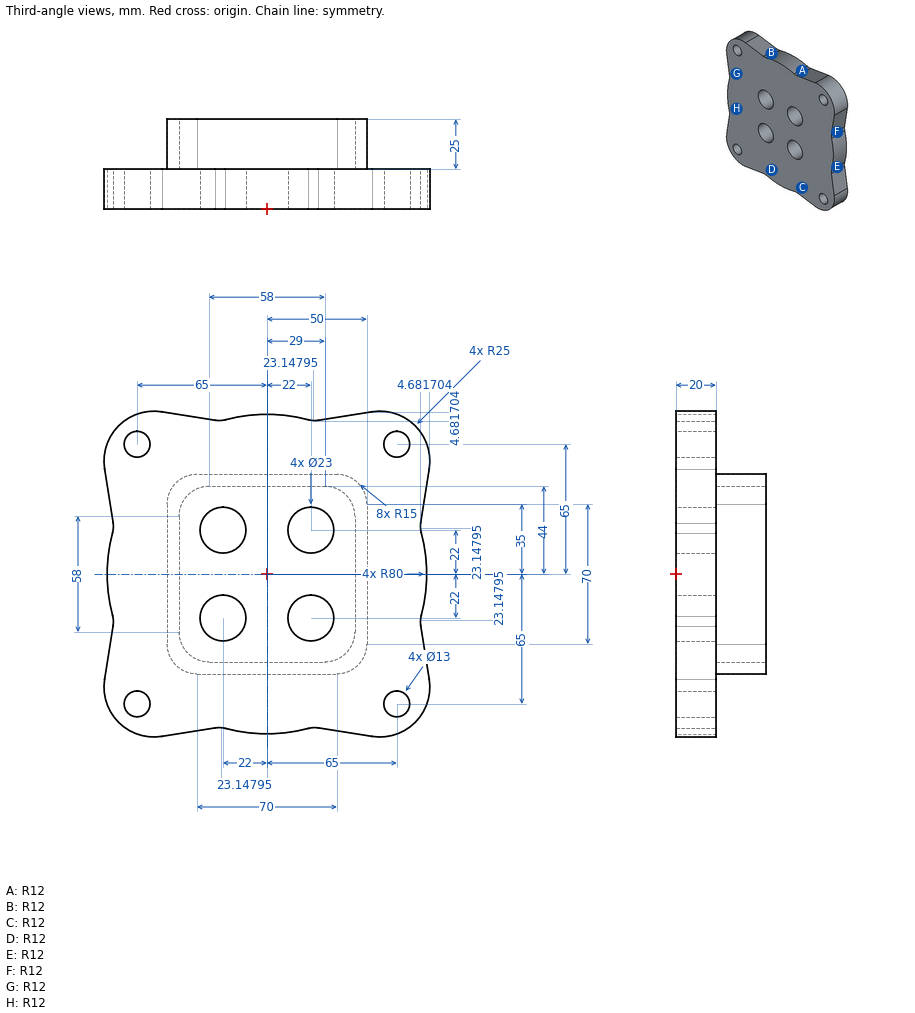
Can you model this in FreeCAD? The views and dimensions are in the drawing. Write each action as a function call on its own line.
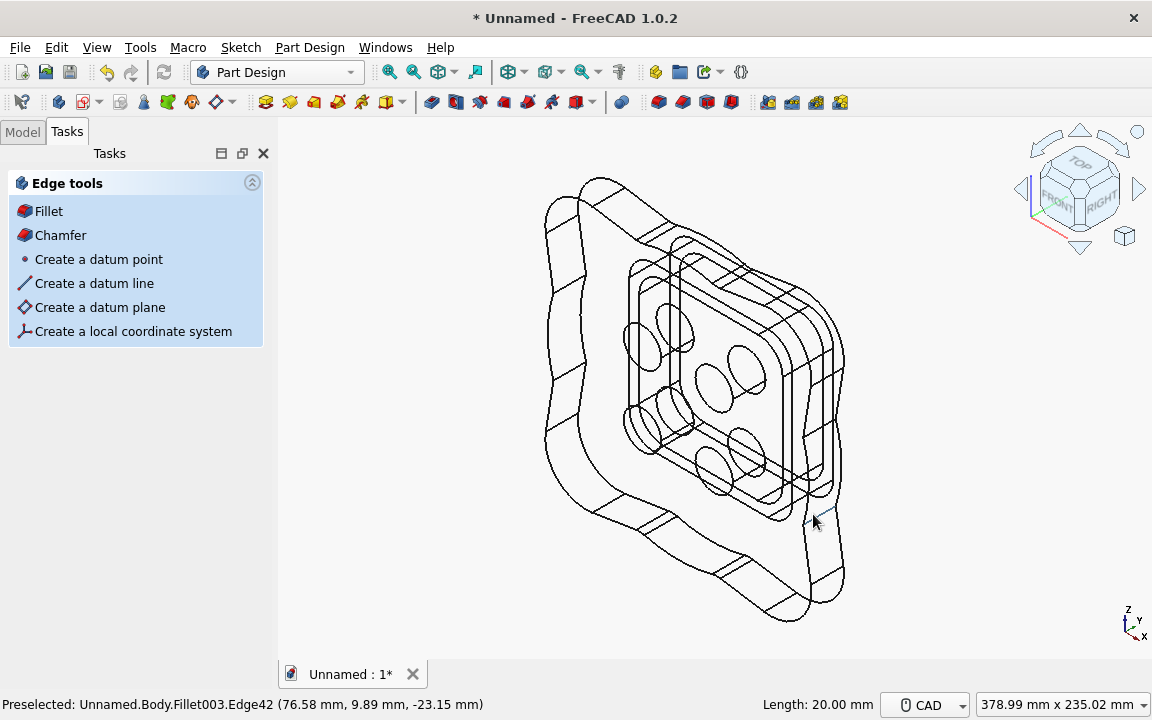
key(v)
key(1)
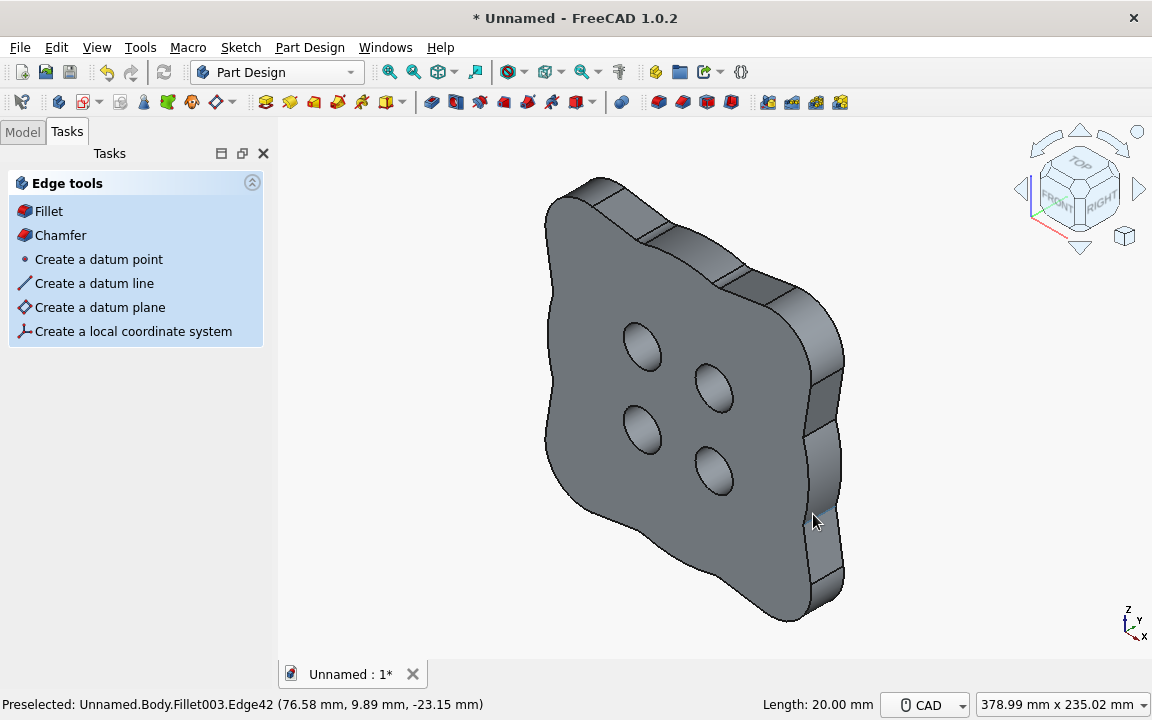
click(660, 102)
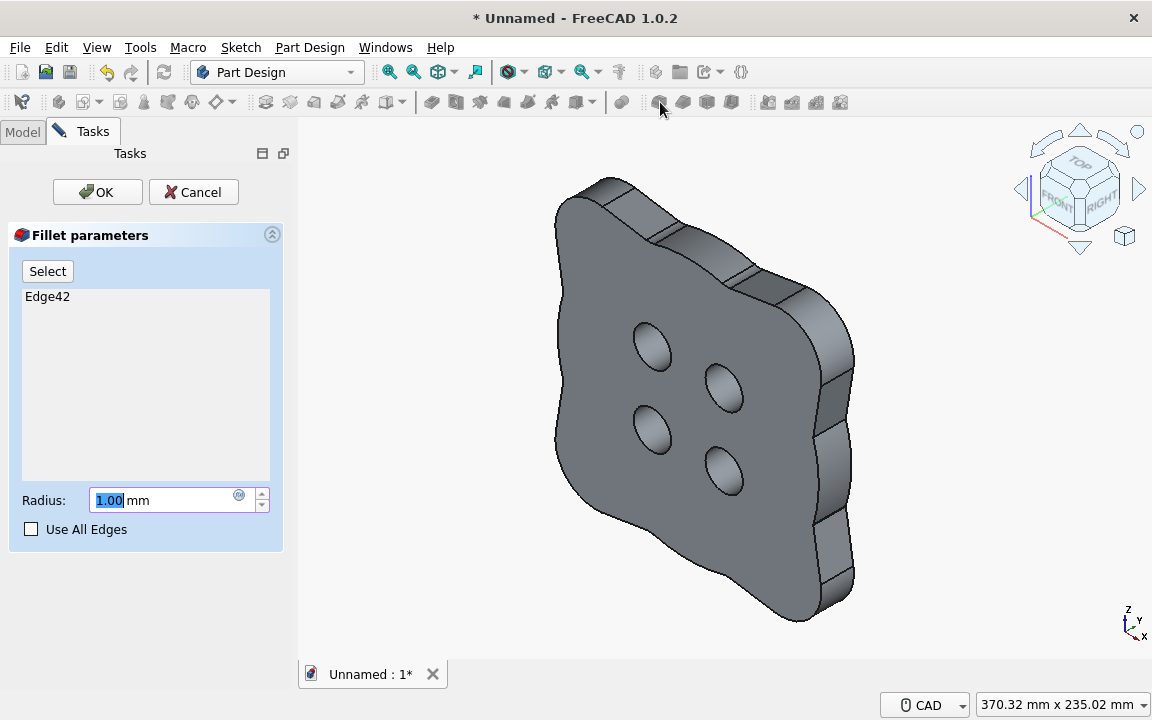
text(12)
key(Tab)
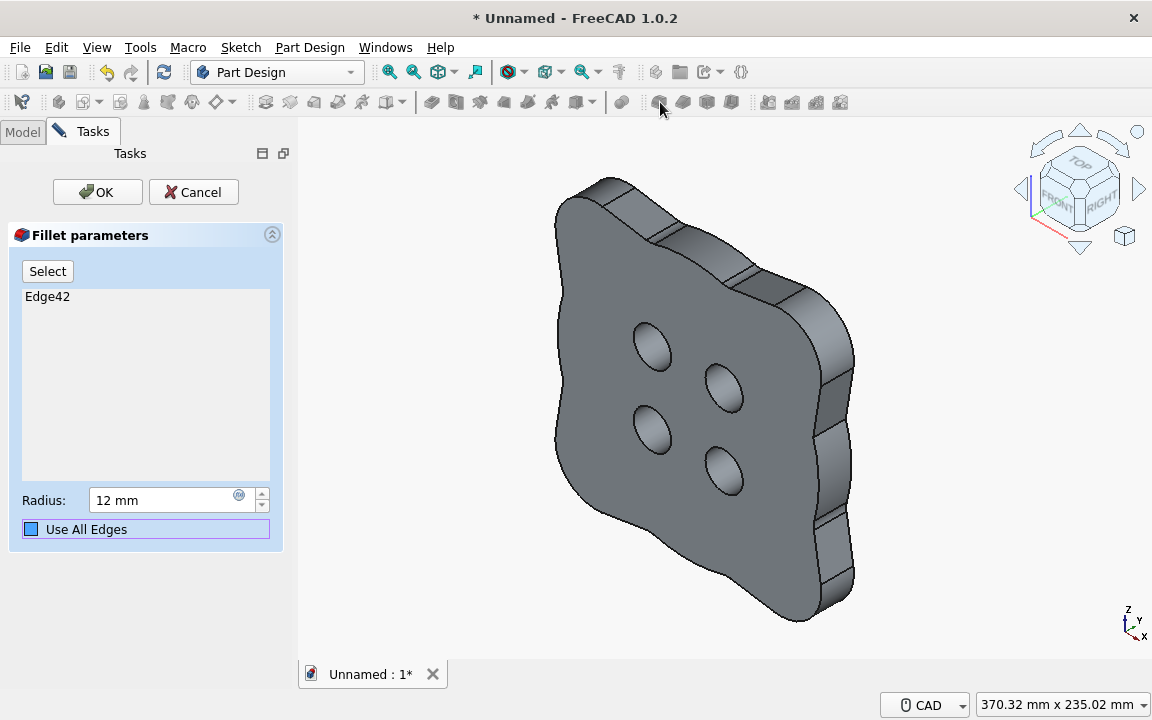
click(98, 192)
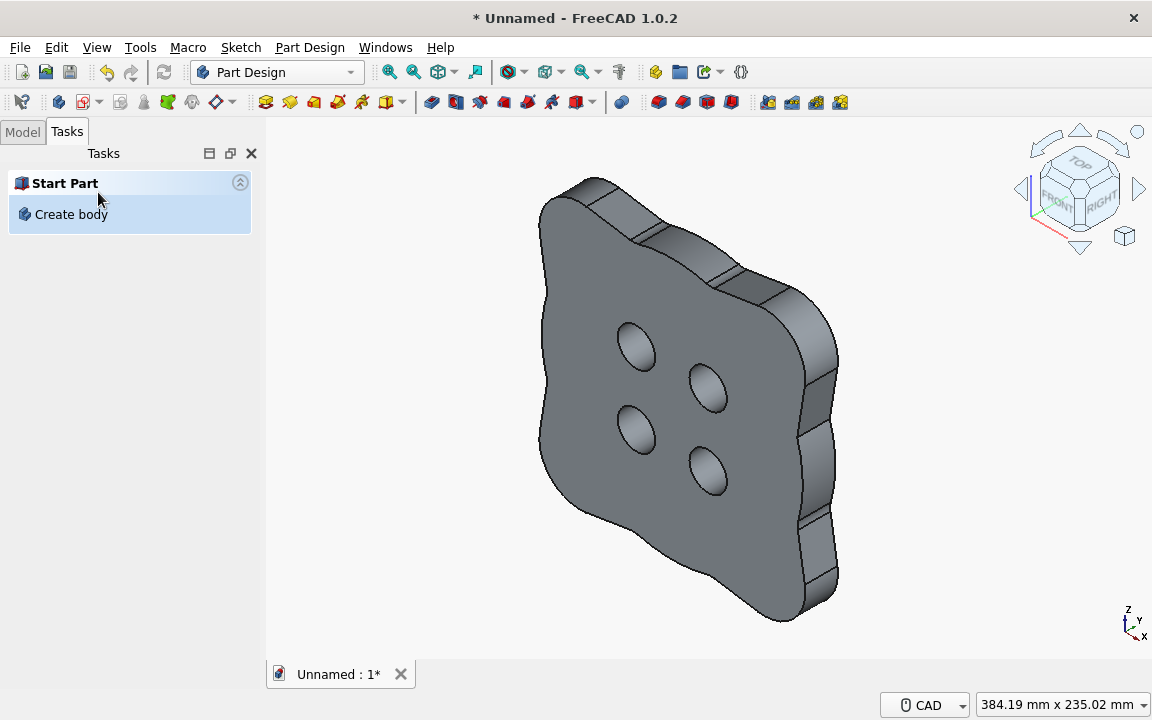
key(2)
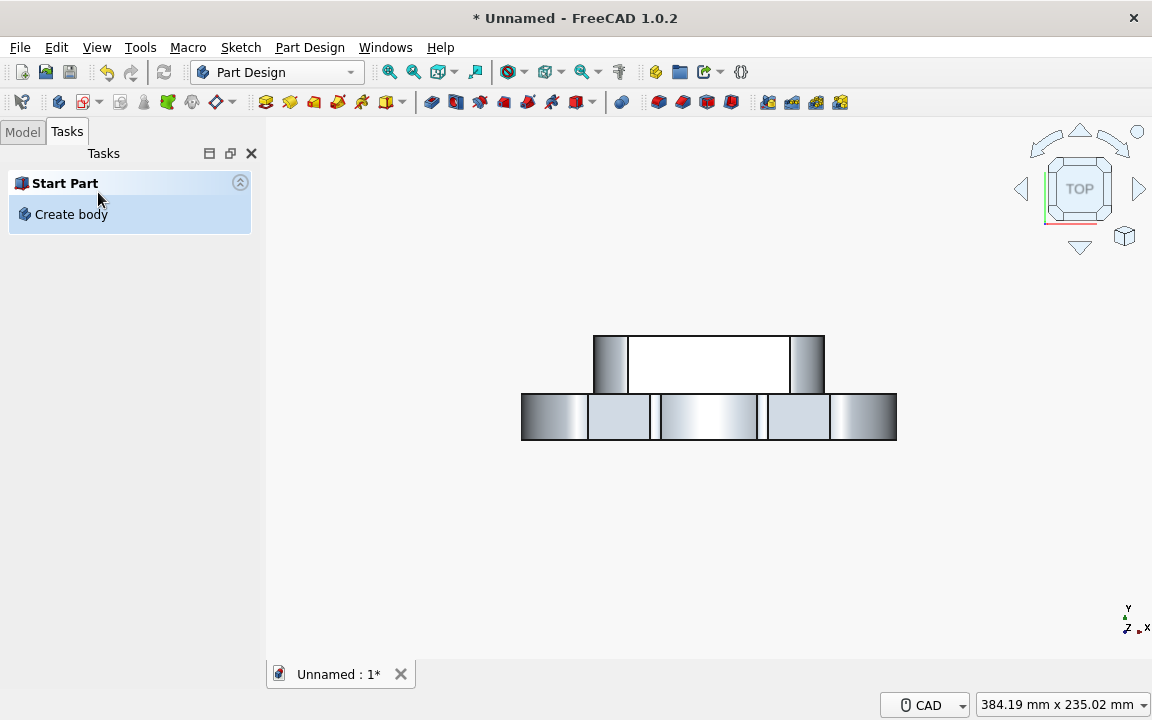
click(390, 72)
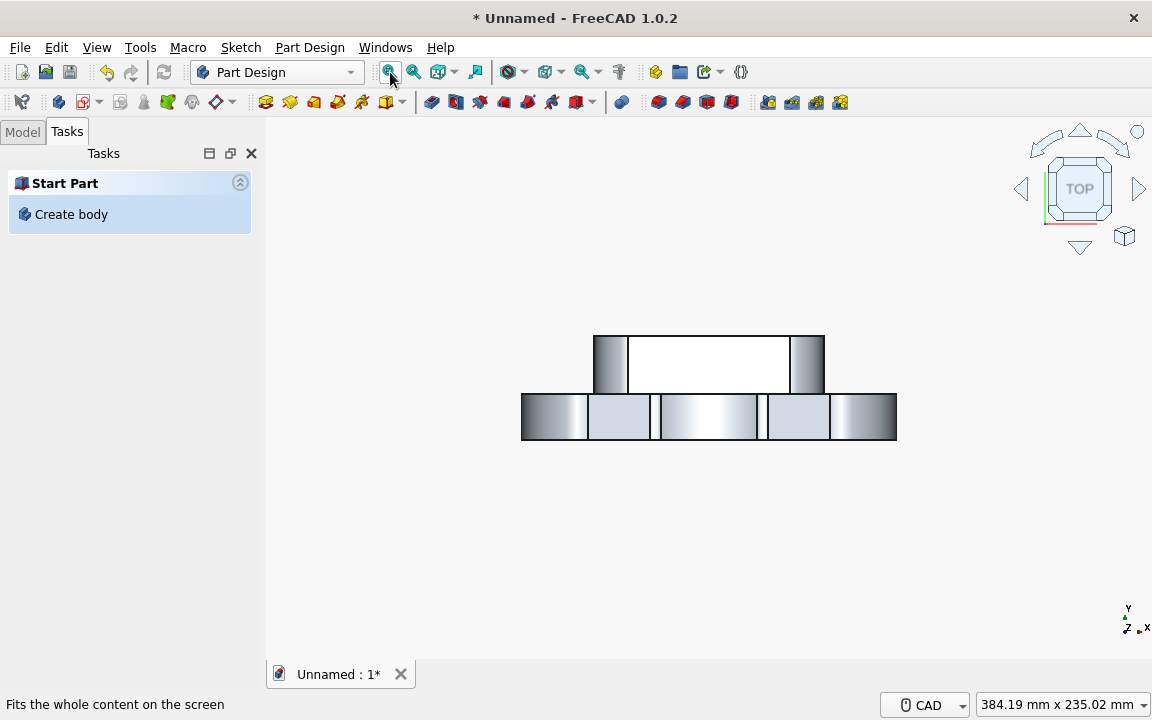
key(0)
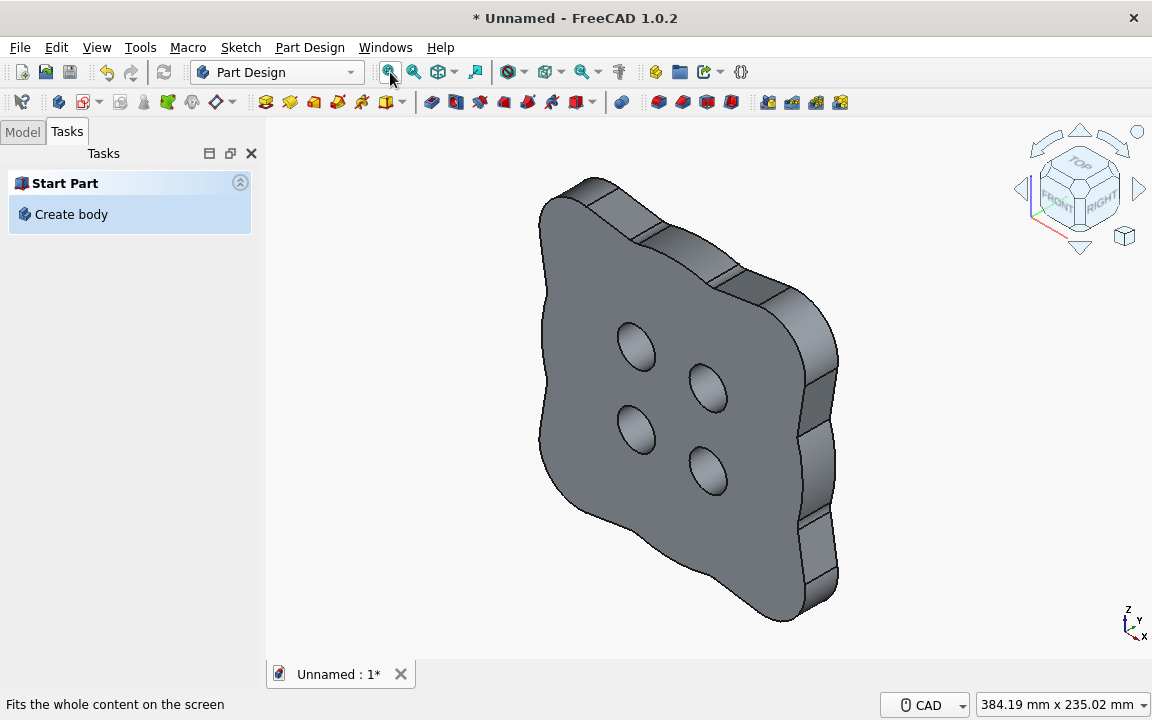
key(1)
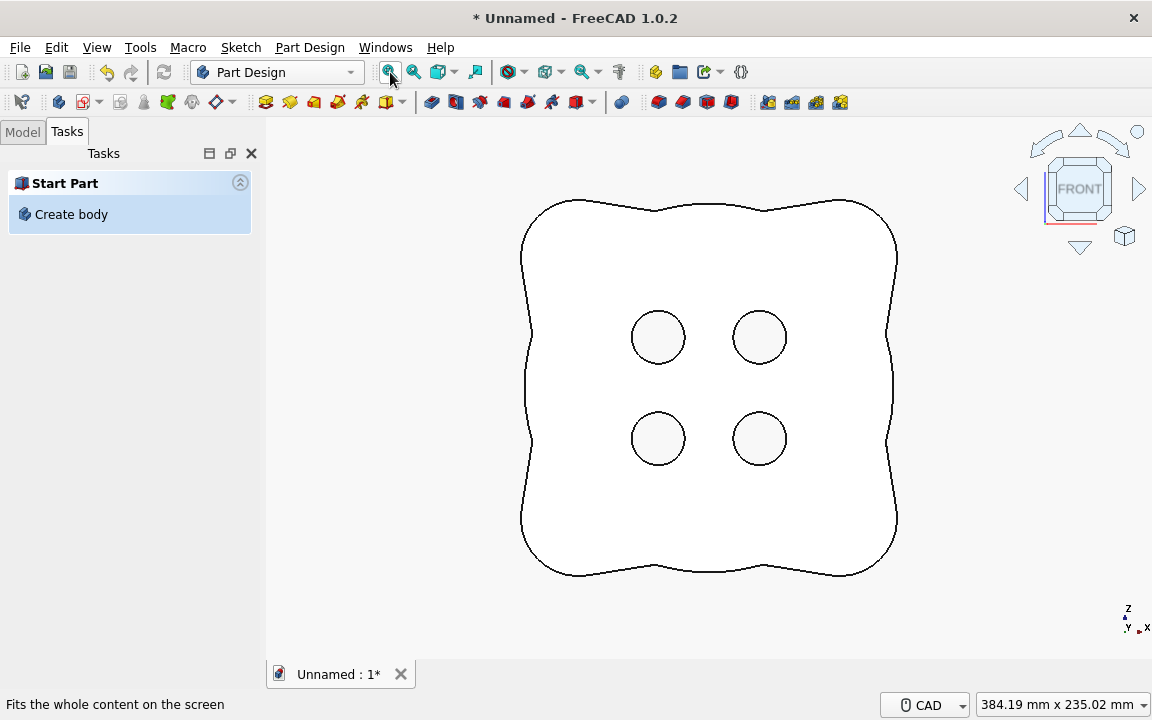
key(3)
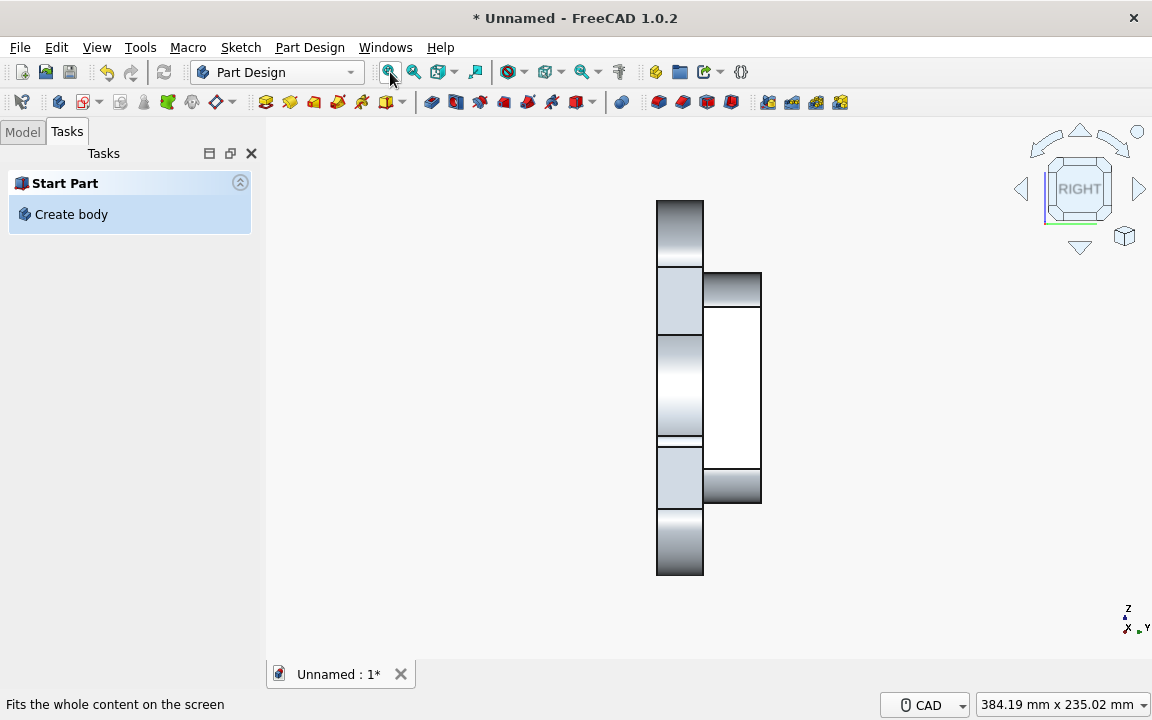
key(5)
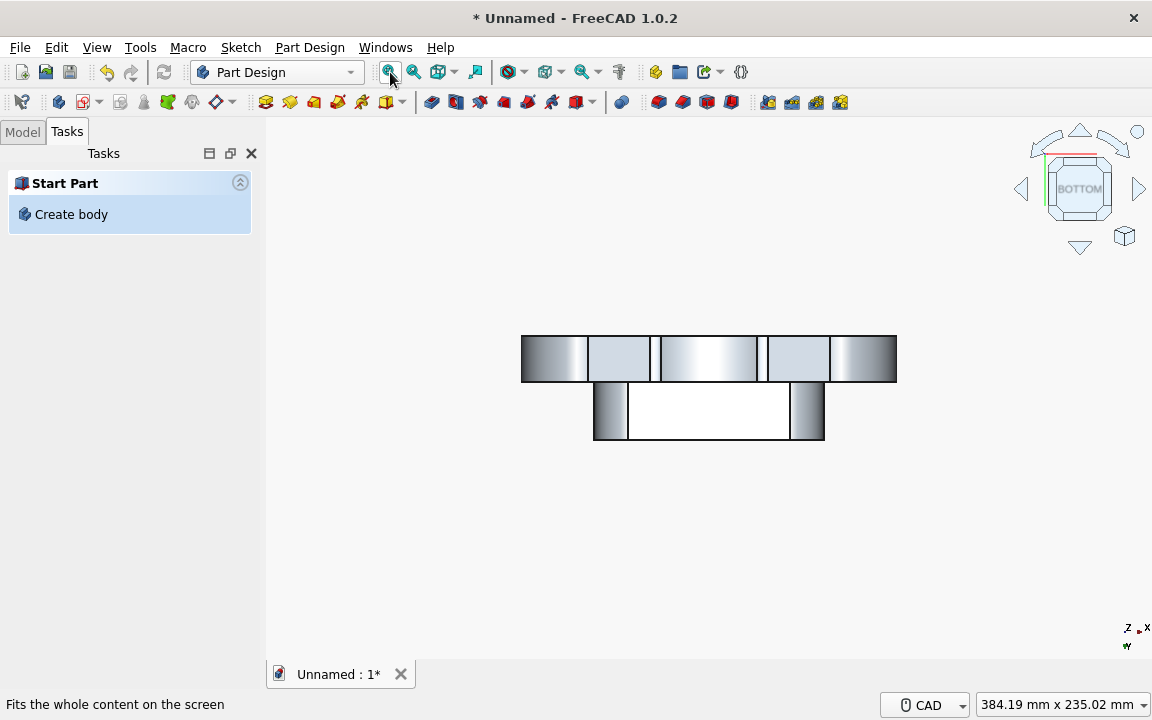
click(390, 72)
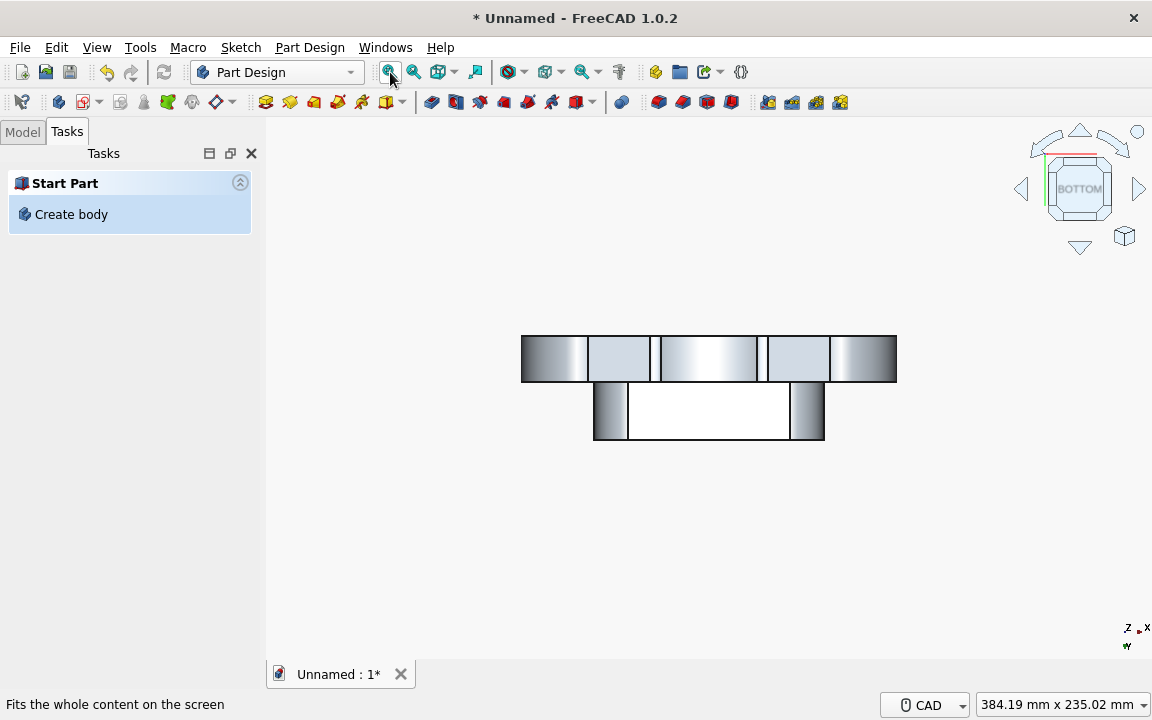
key(4)